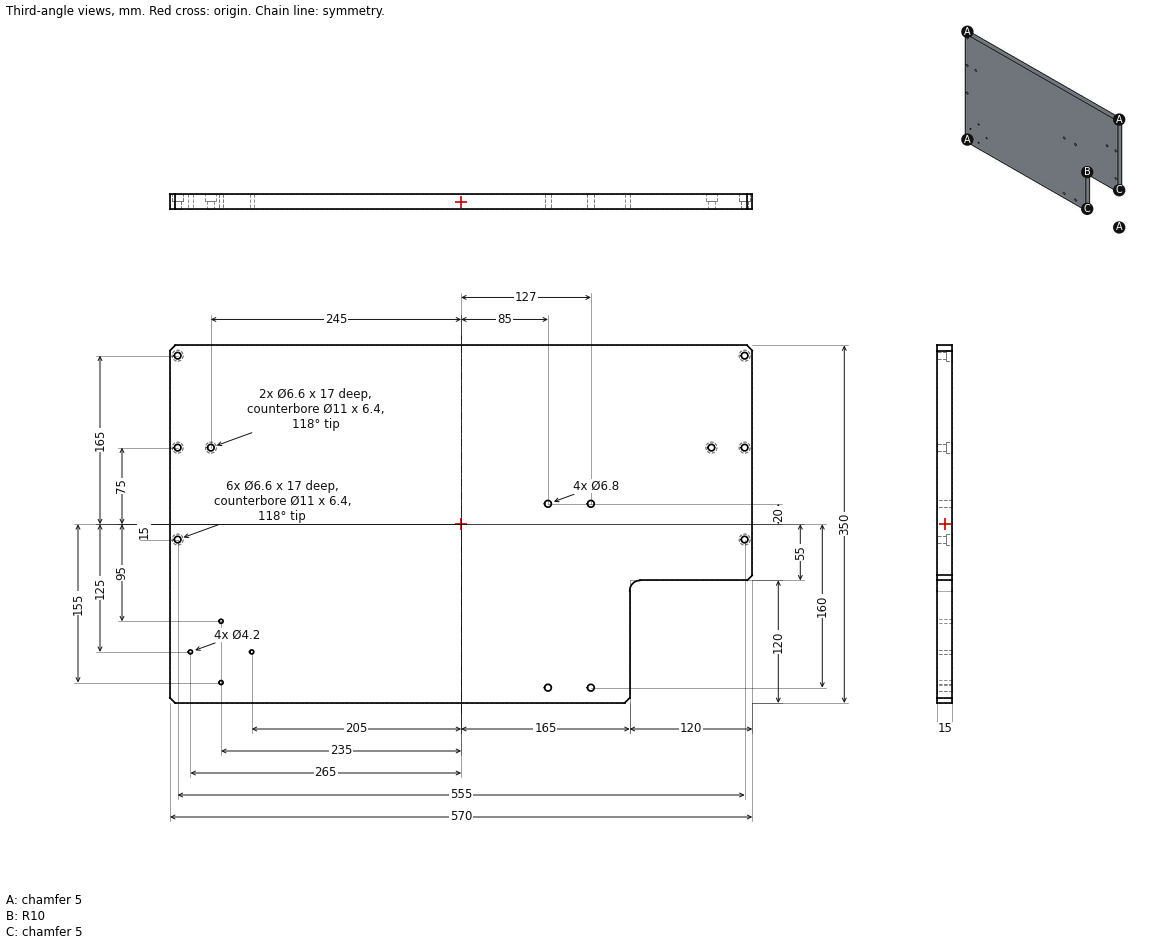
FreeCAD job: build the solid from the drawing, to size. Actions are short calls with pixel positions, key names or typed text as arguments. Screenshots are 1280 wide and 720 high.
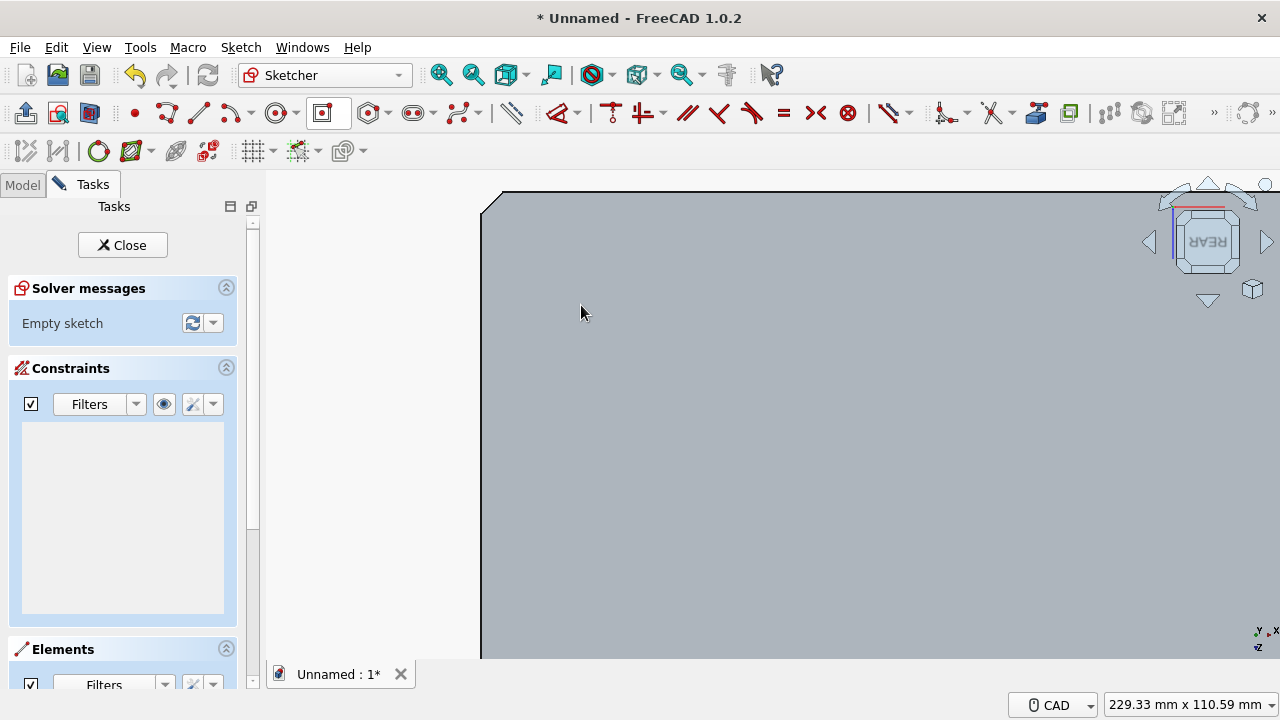
click(276, 114)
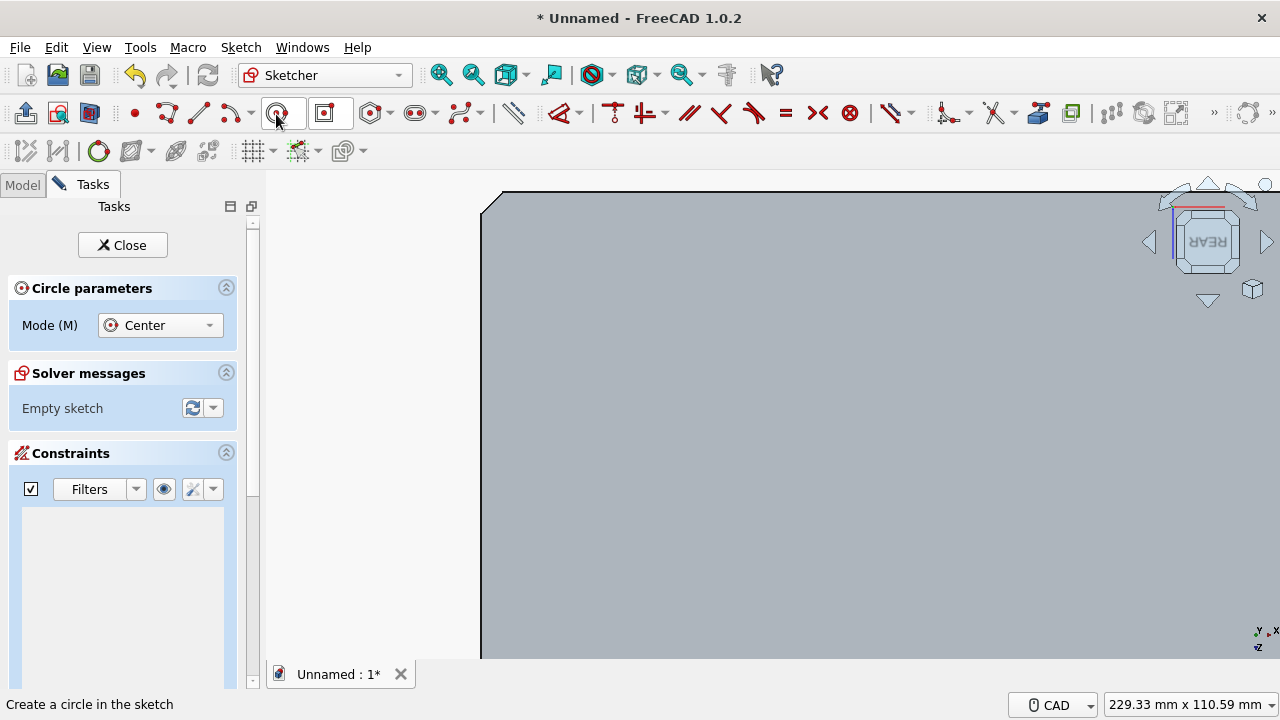
scroll(569, 413, up, 5)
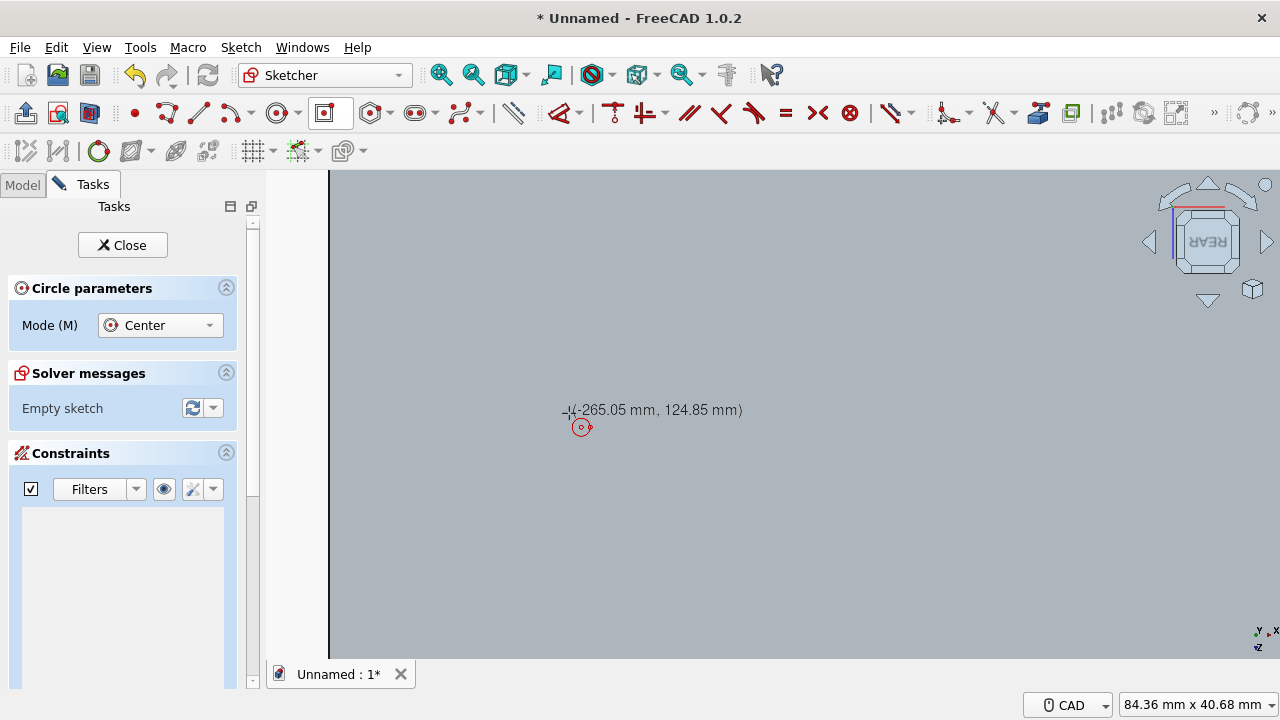
click(569, 413)
move(587, 395)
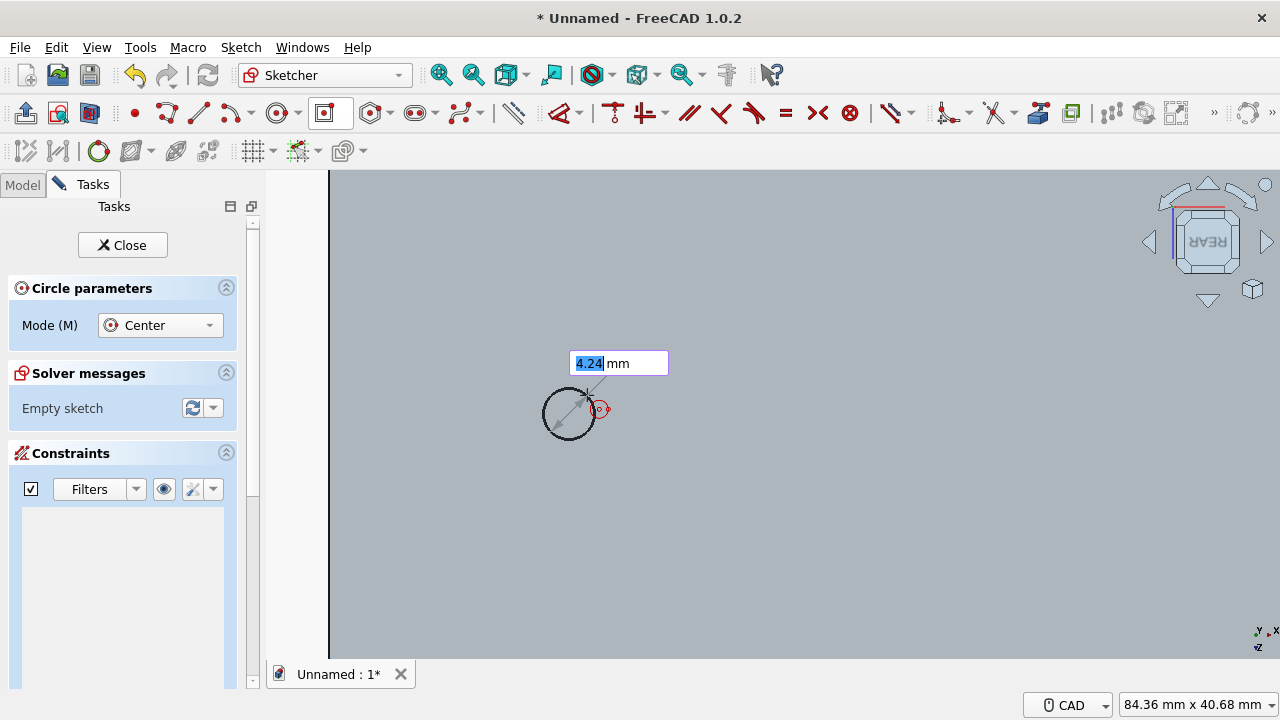
text(4.2)
key(Return)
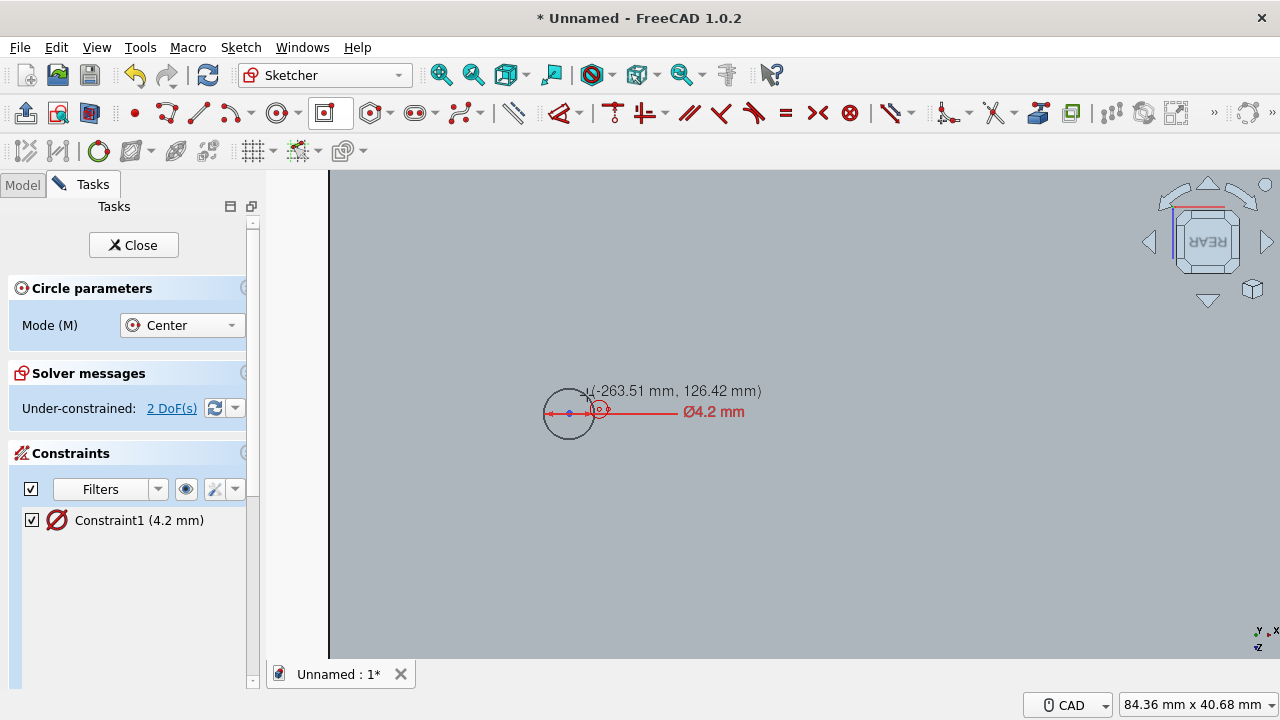
scroll(573, 415, down, 5)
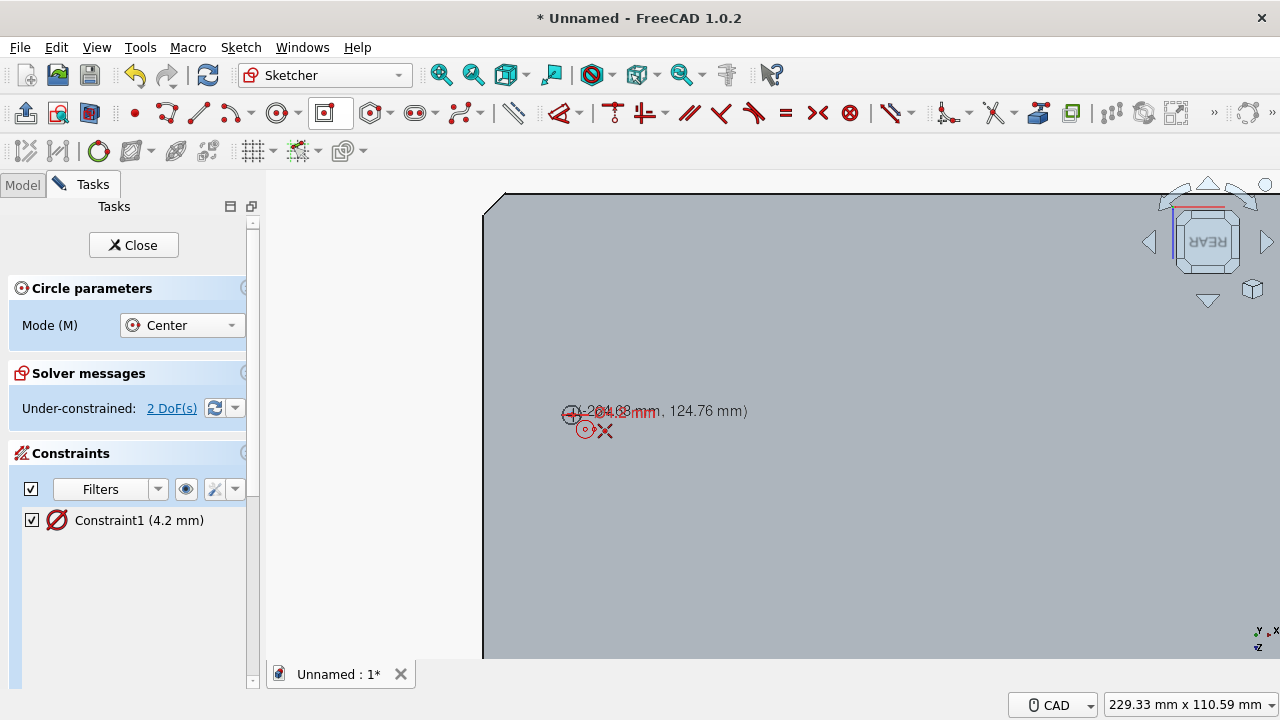
scroll(704, 547, up, 5)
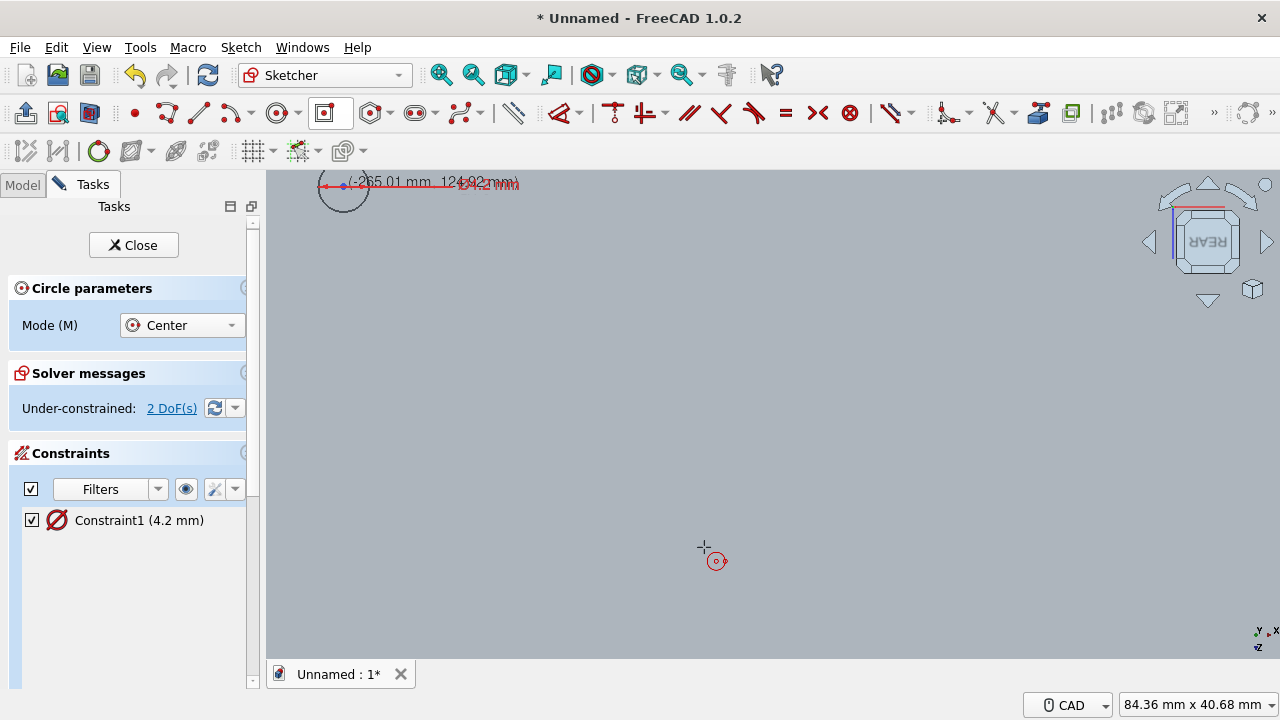
click(704, 546)
move(722, 529)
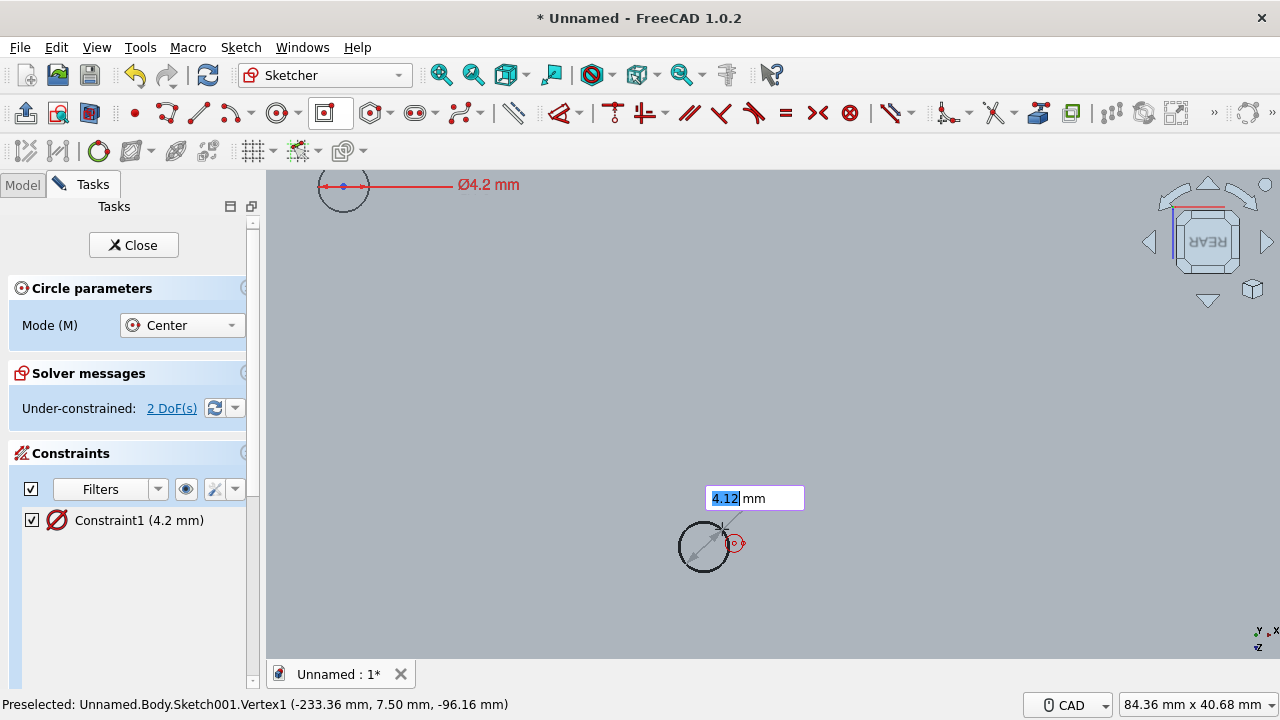
text(4.2)
key(Return)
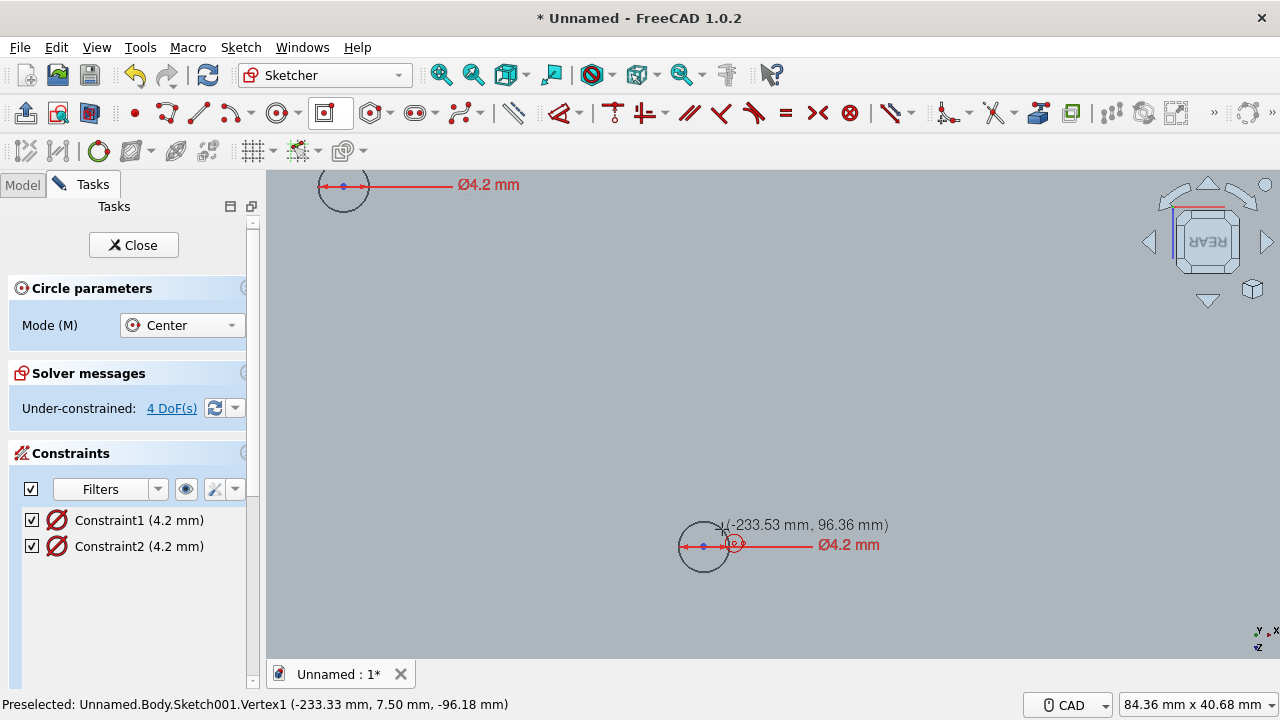
scroll(705, 548, down, 5)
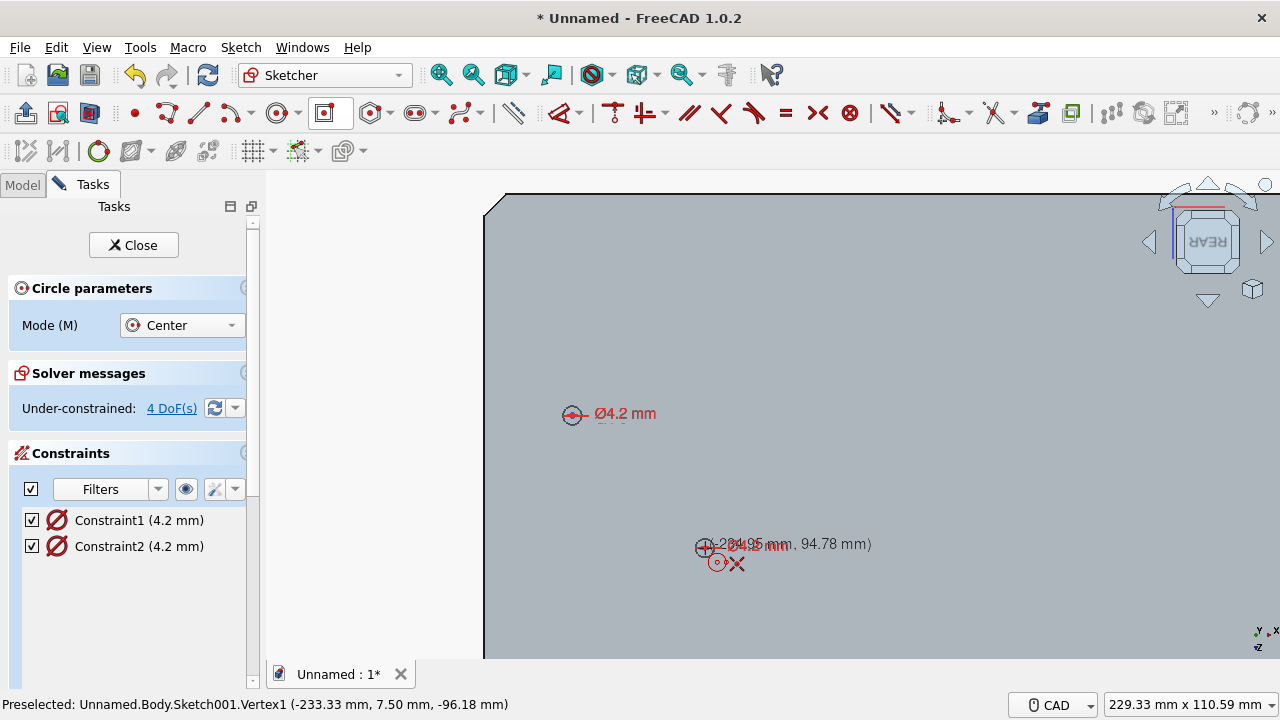
scroll(705, 283, up, 5)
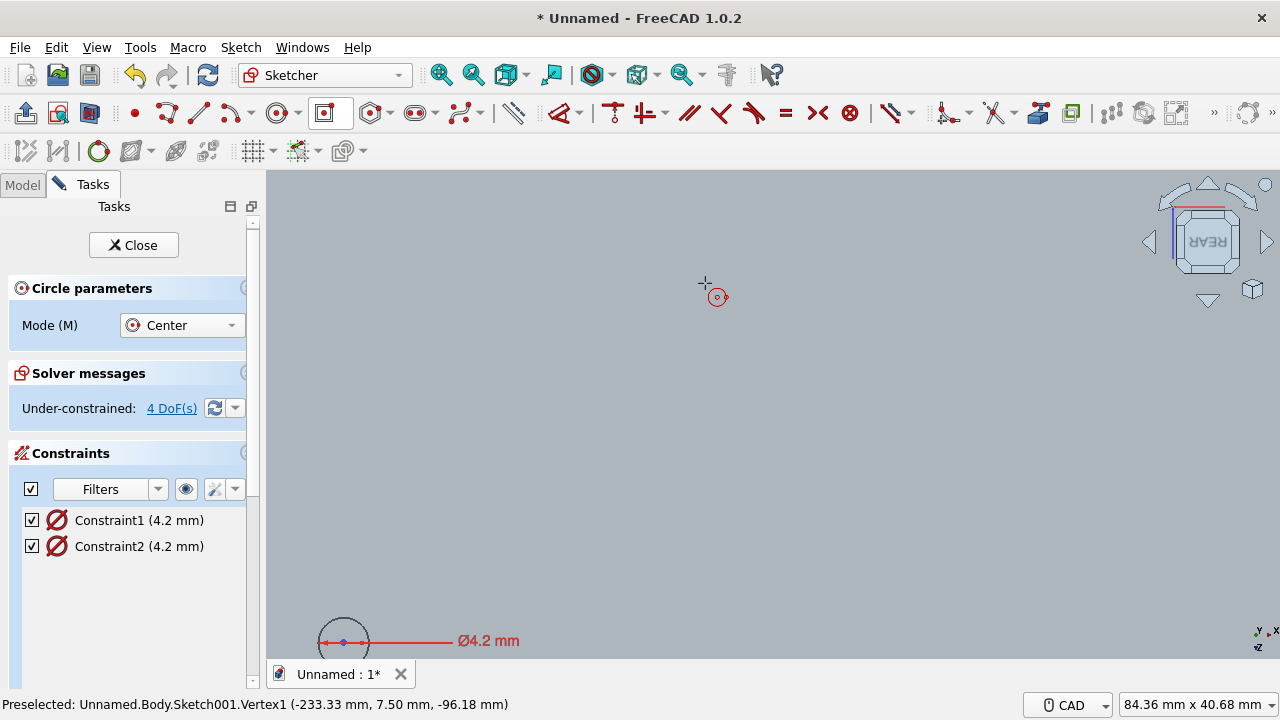
click(704, 281)
move(722, 264)